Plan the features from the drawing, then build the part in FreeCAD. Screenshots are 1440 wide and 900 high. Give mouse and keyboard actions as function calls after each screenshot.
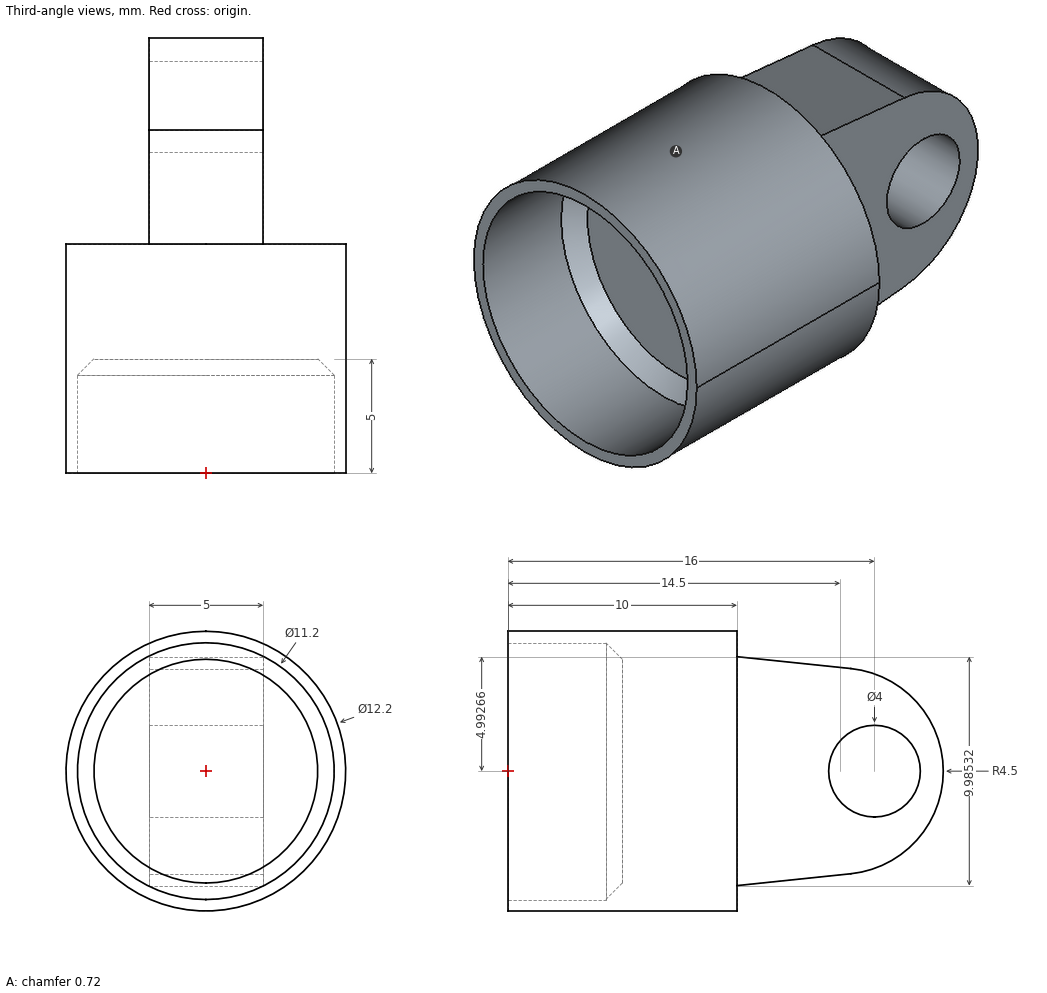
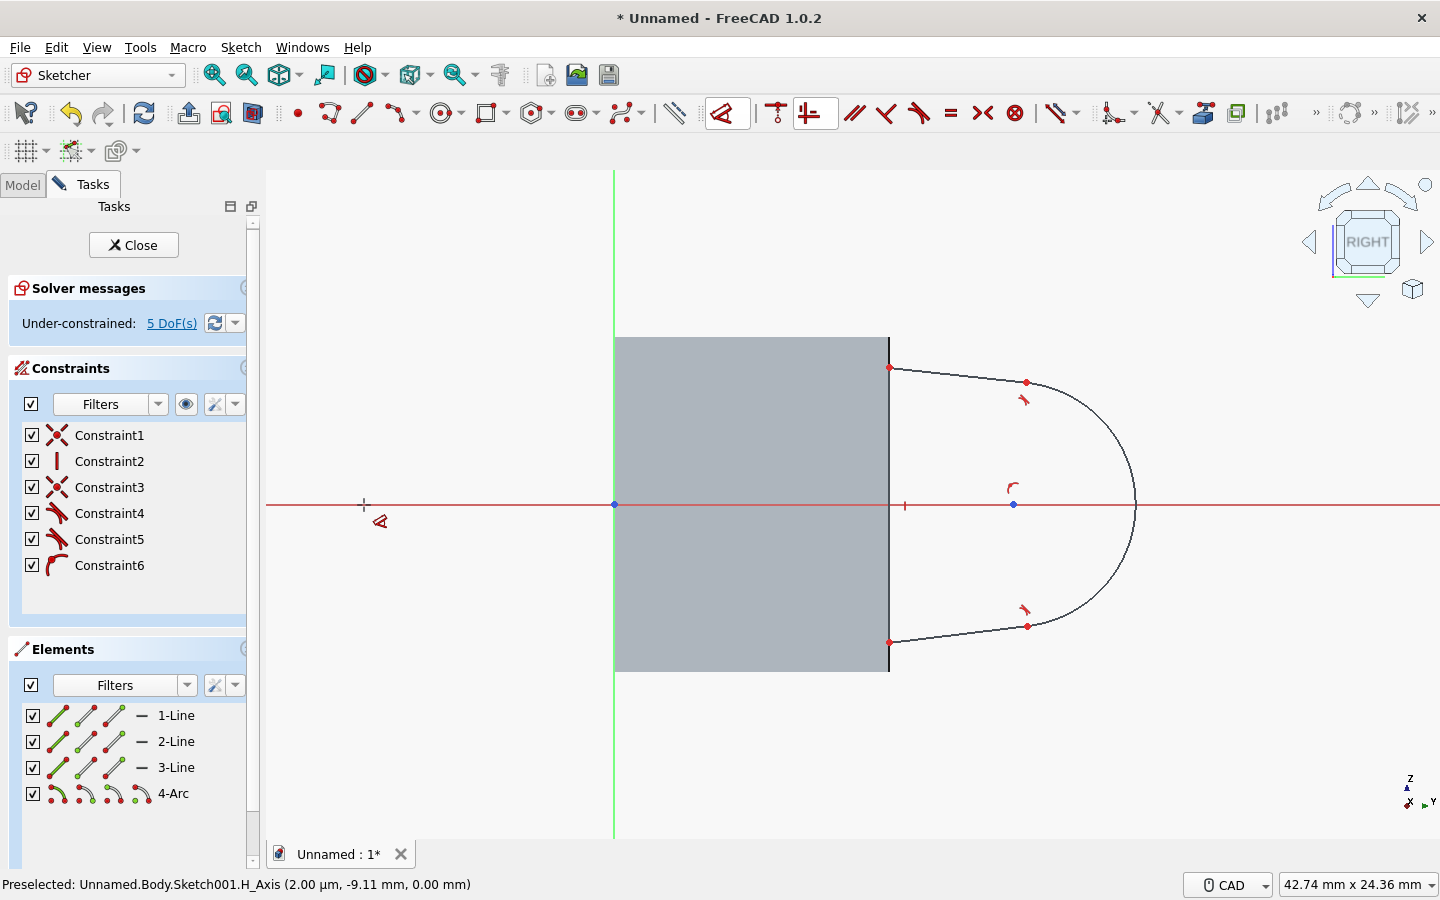
click(1116, 571)
click(1143, 588)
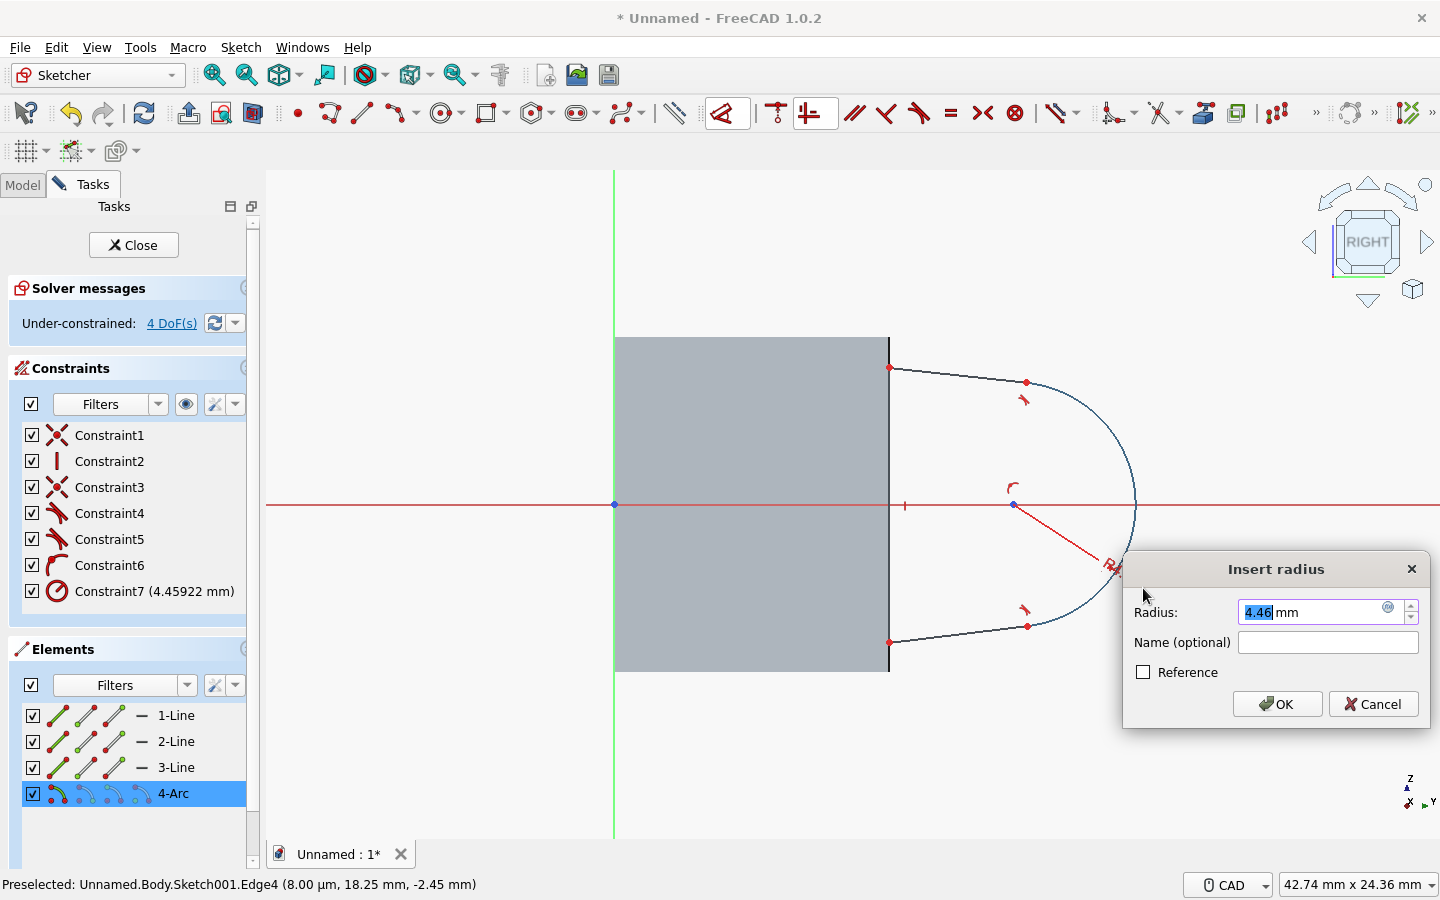
text(4.5)
key(Return)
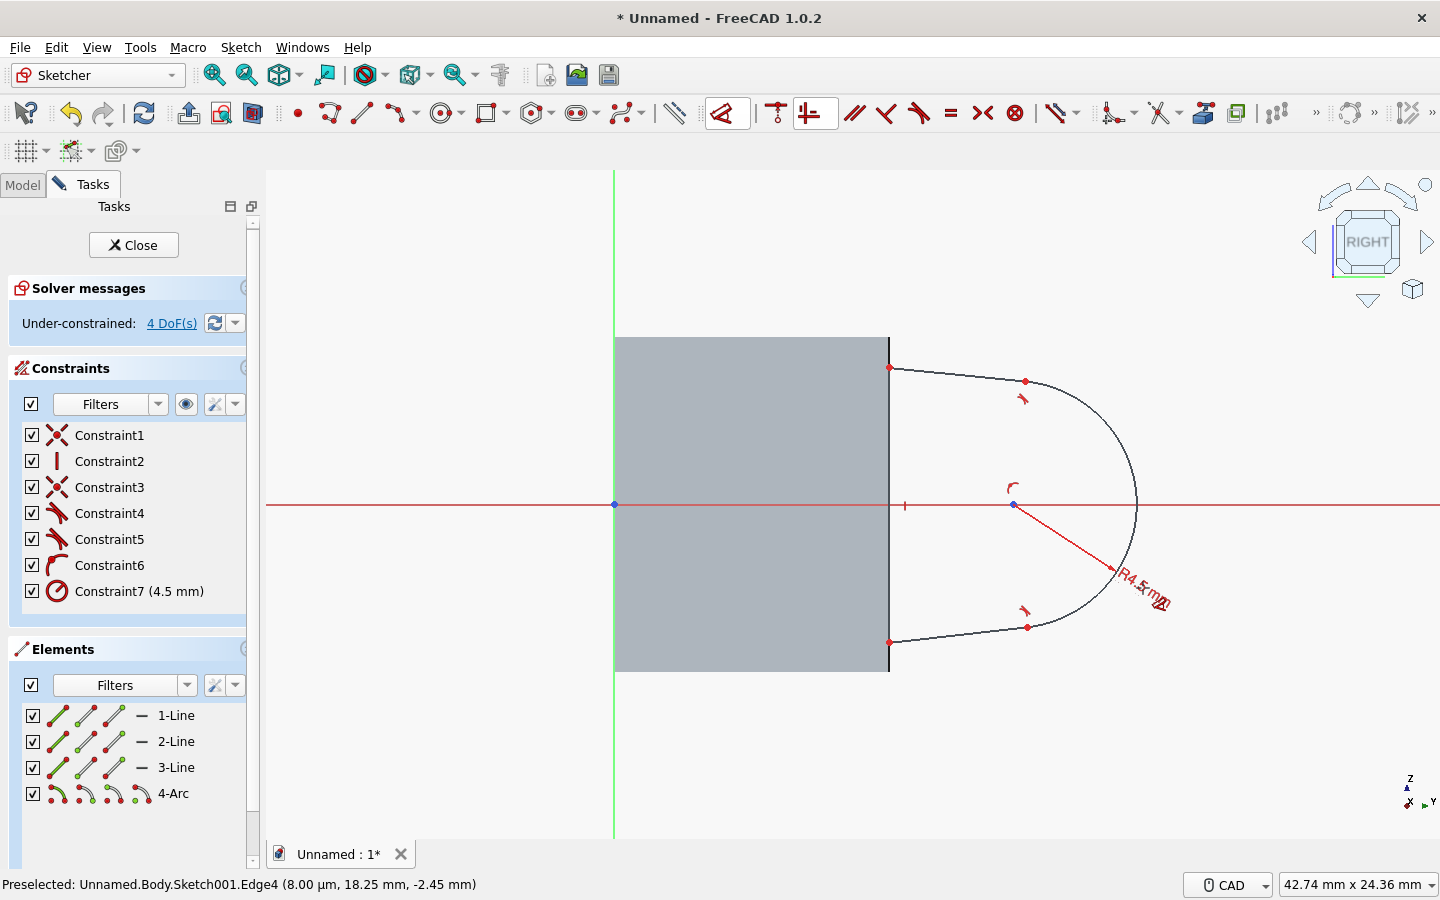
click(889, 368)
click(752, 334)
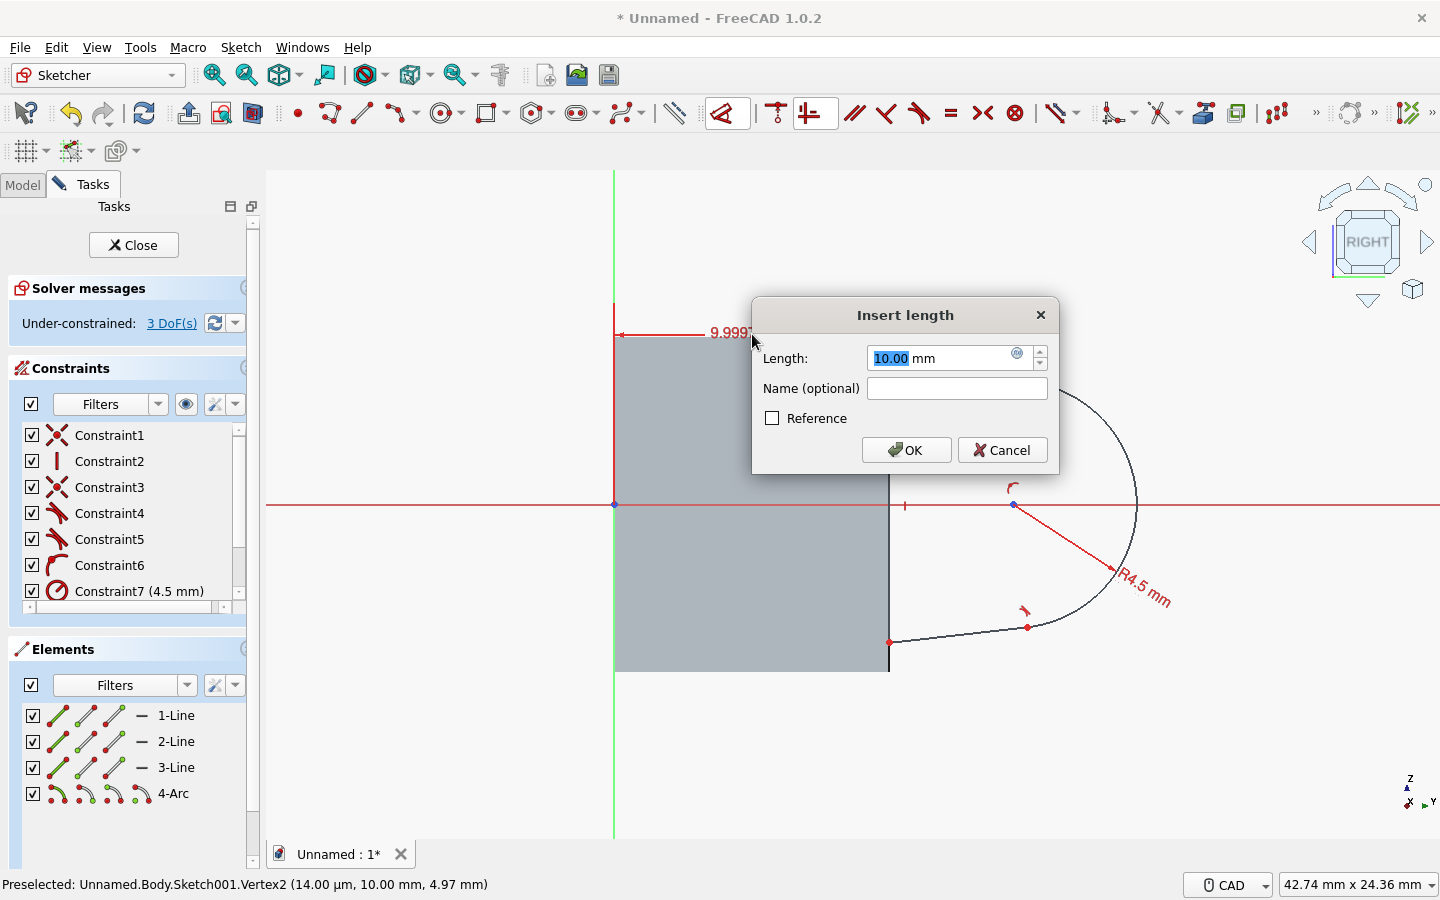
text(10)
key(Return)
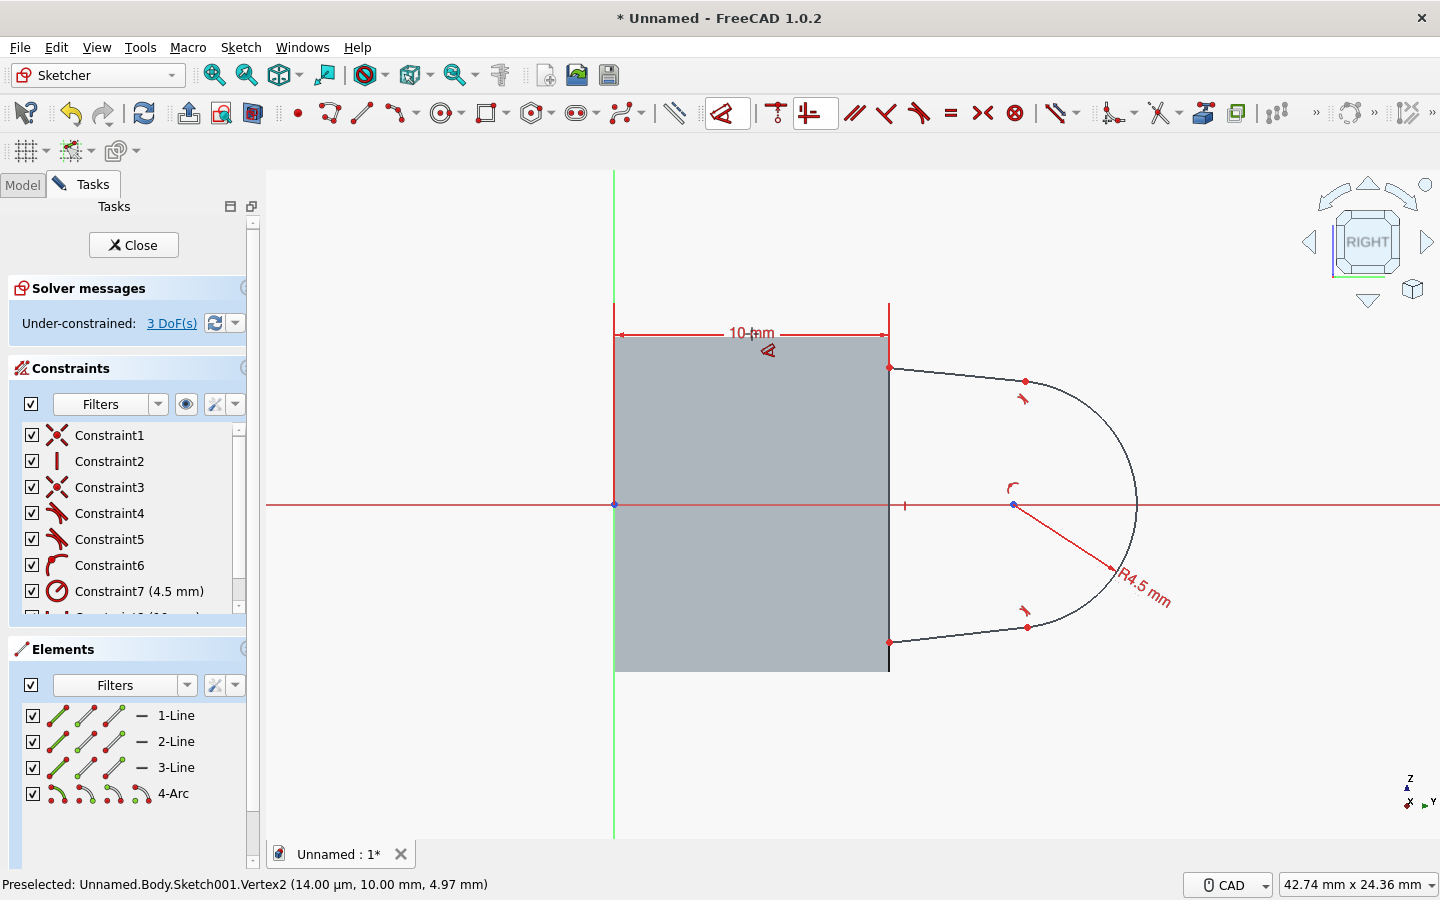
click(1013, 505)
click(814, 539)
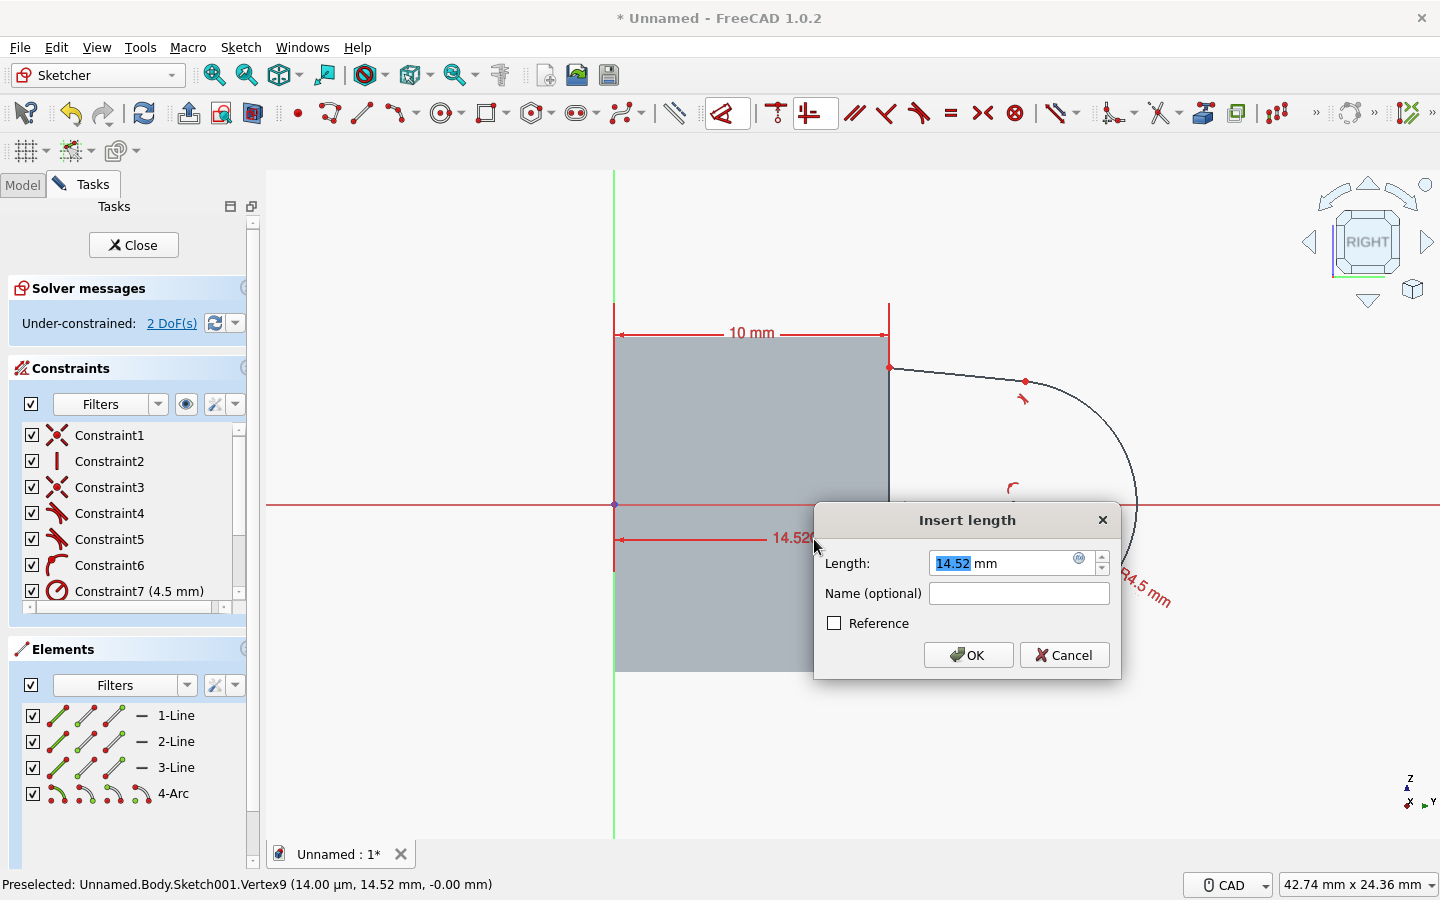
text(14.5)
key(Return)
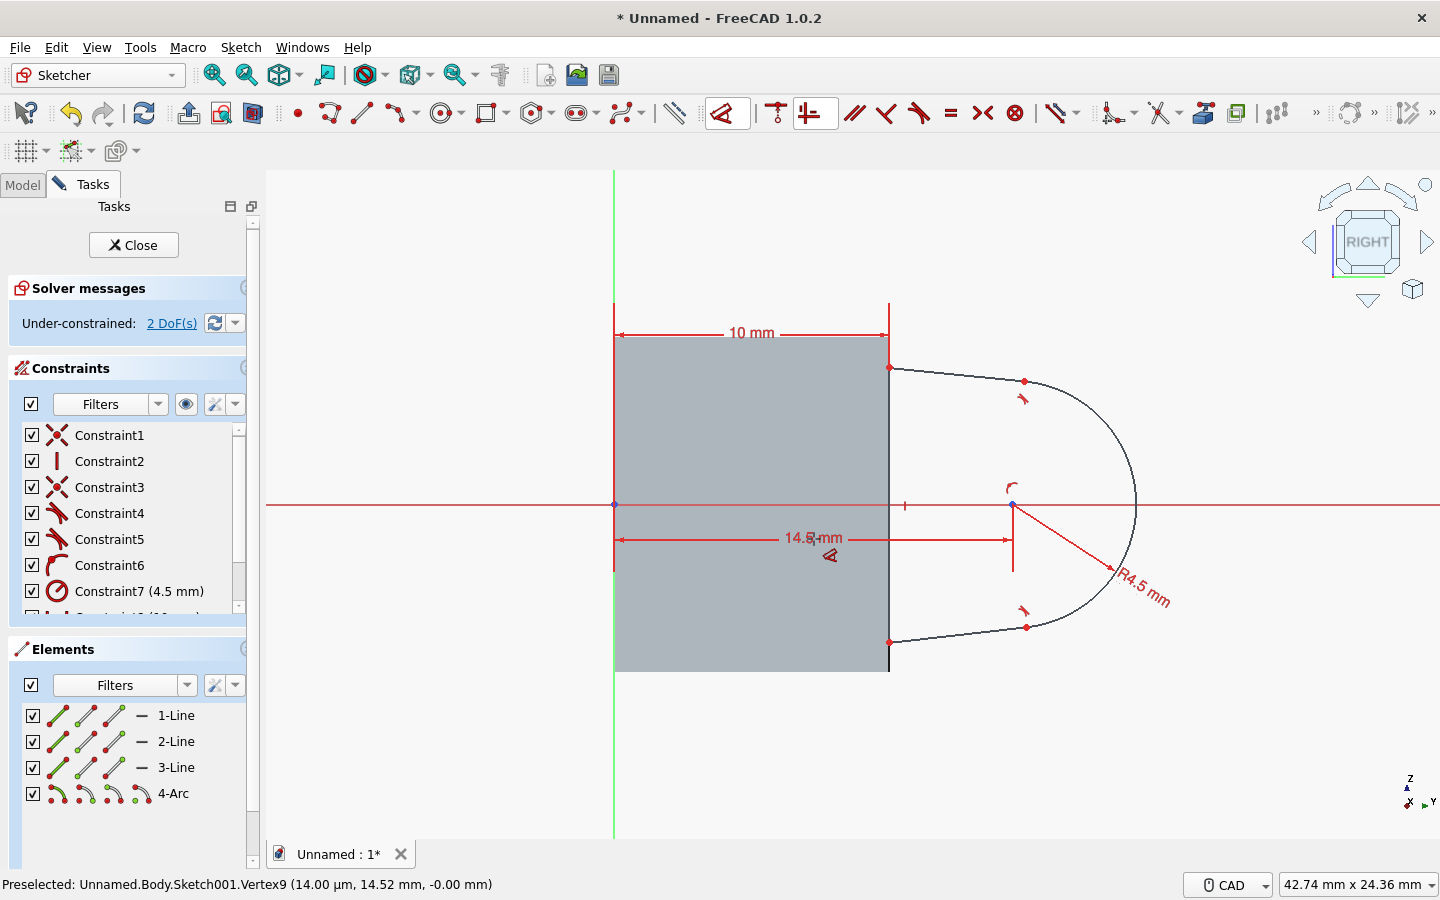
click(889, 450)
click(923, 442)